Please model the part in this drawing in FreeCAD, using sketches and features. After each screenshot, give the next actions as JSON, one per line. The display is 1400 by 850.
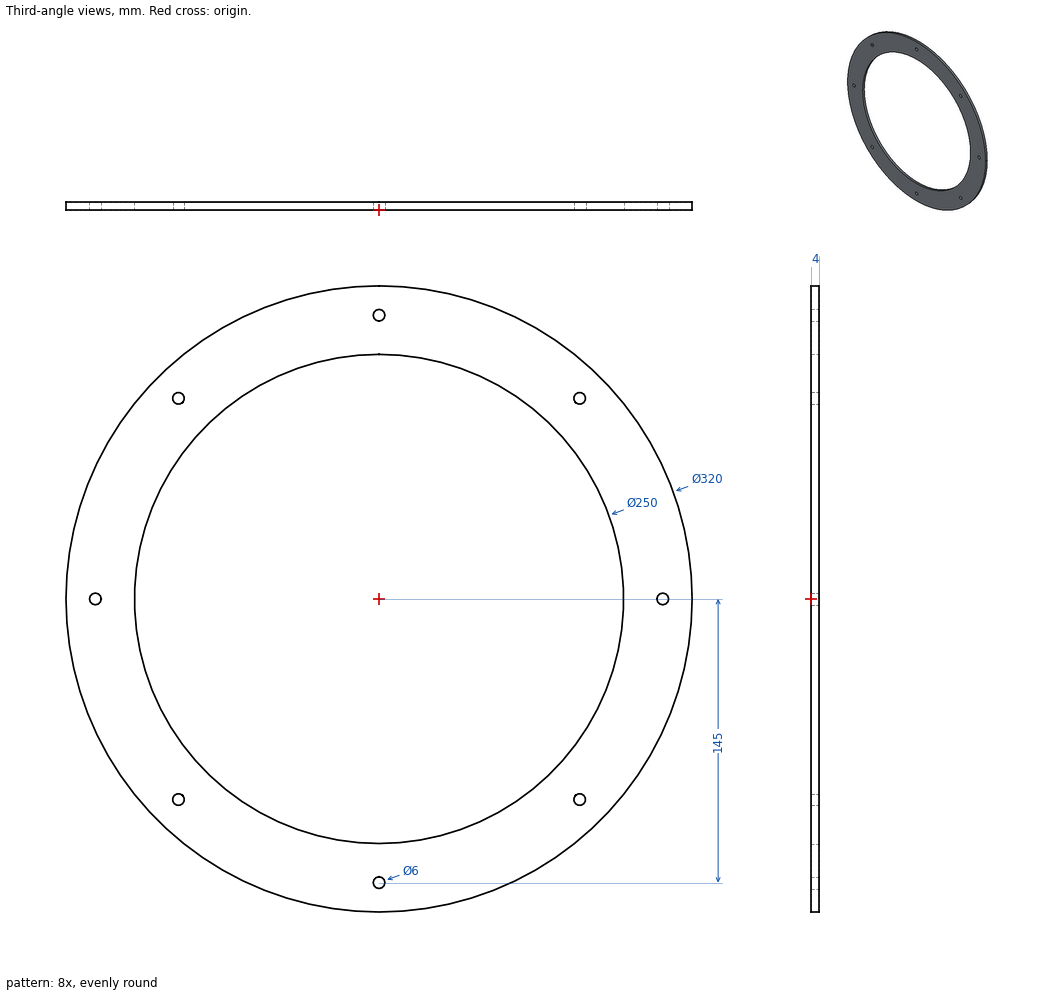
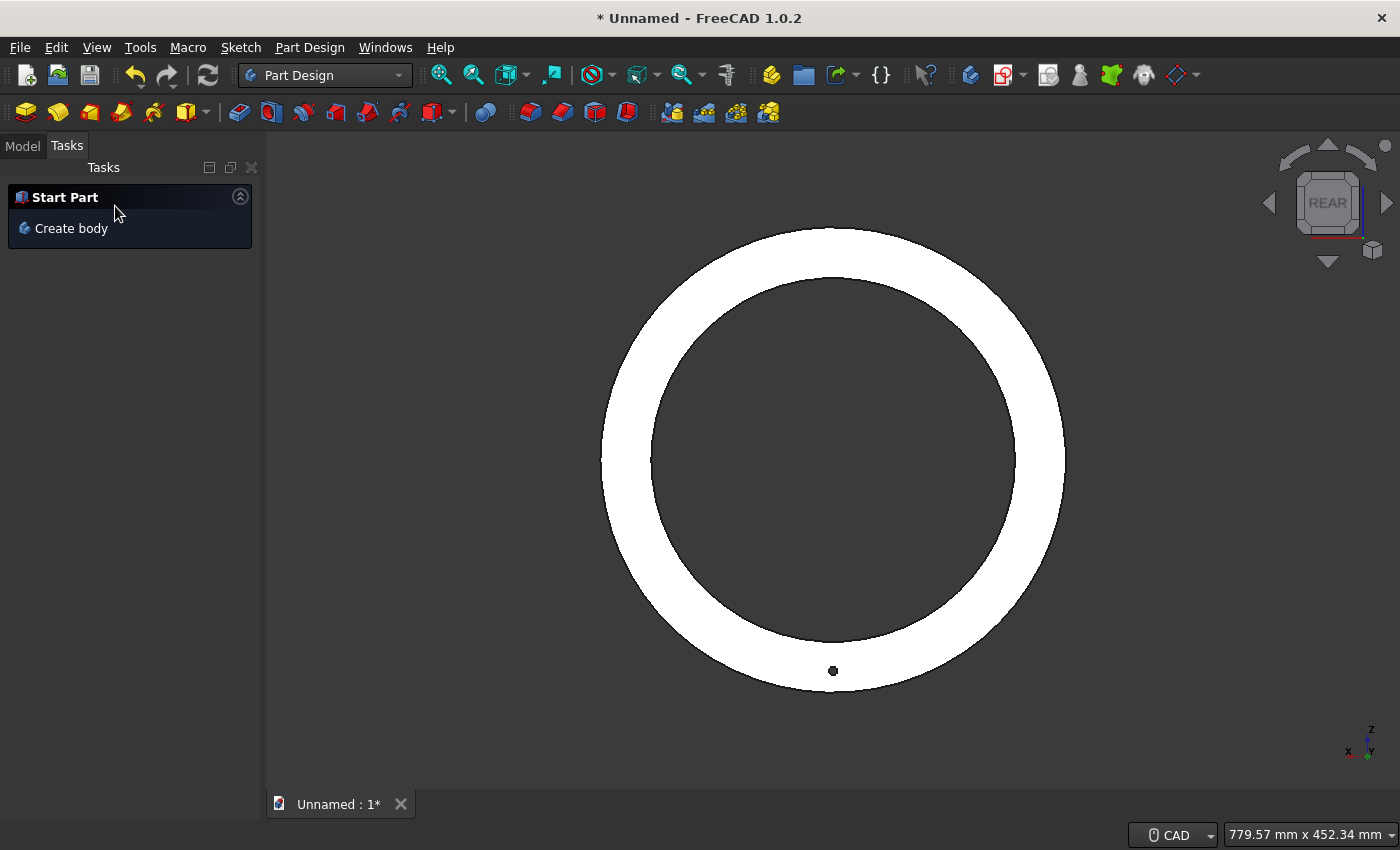
{"action": "left_click", "coordinate": [23, 145]}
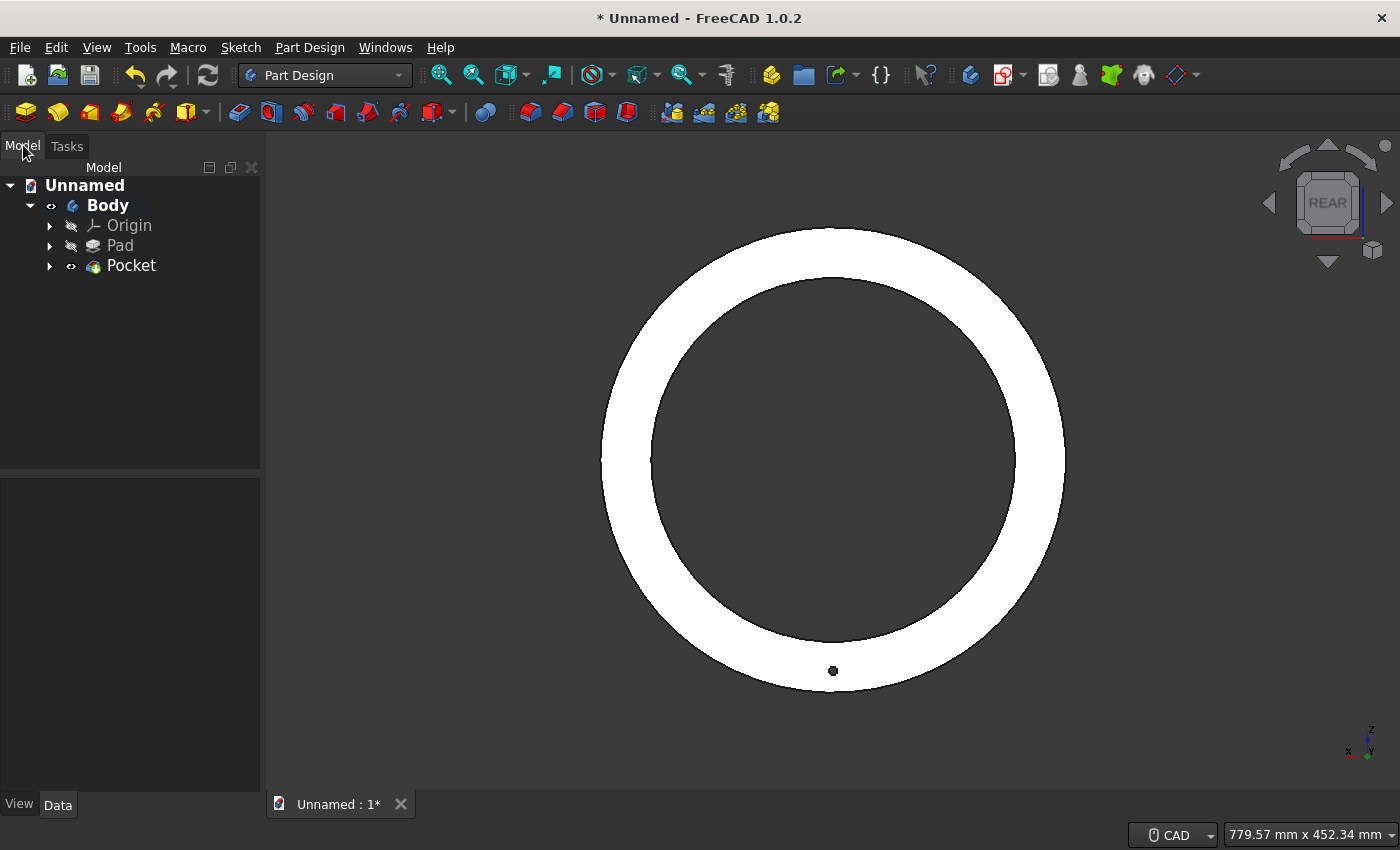
{"action": "left_click", "coordinate": [116, 266]}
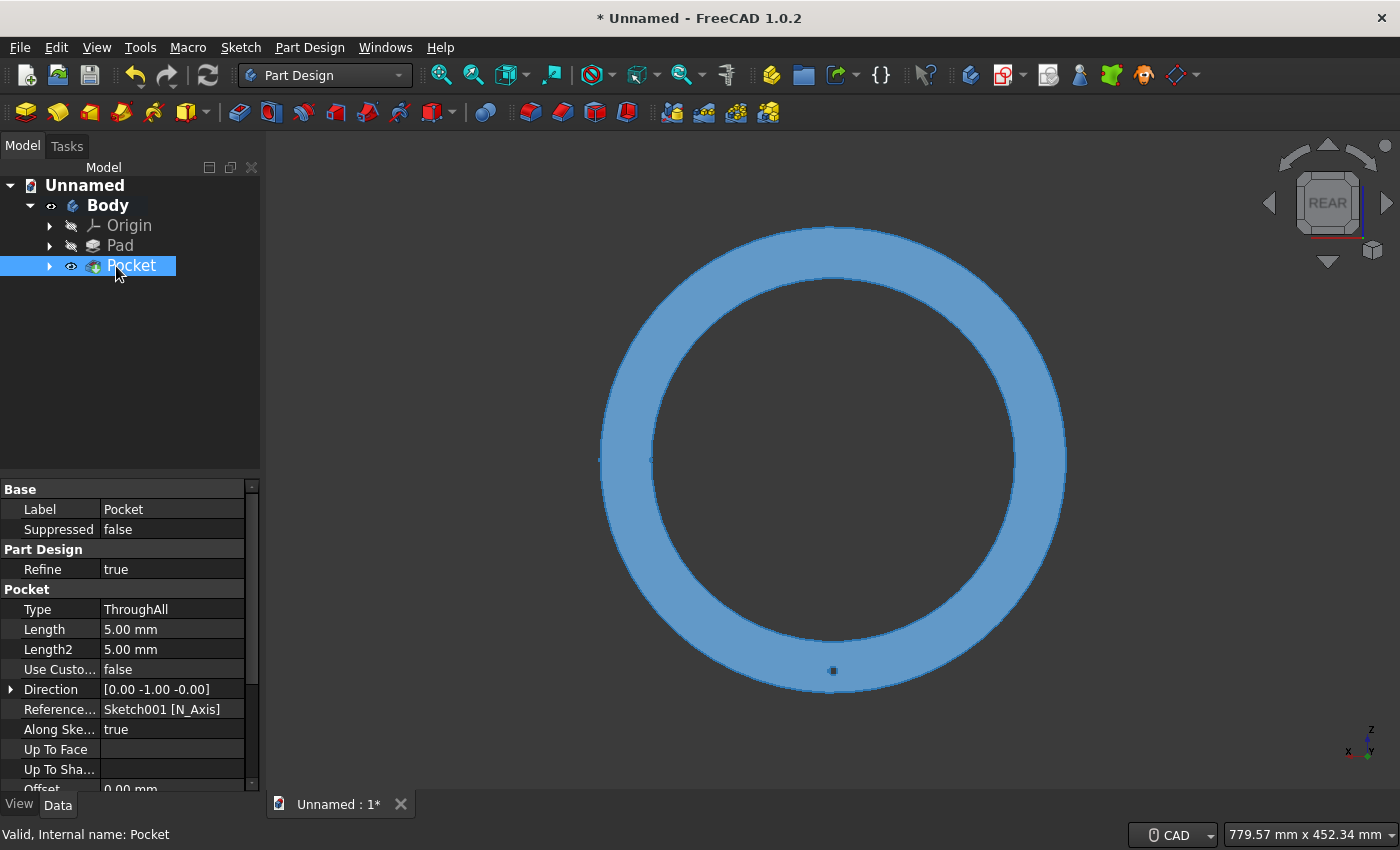
{"action": "left_click", "coordinate": [736, 112]}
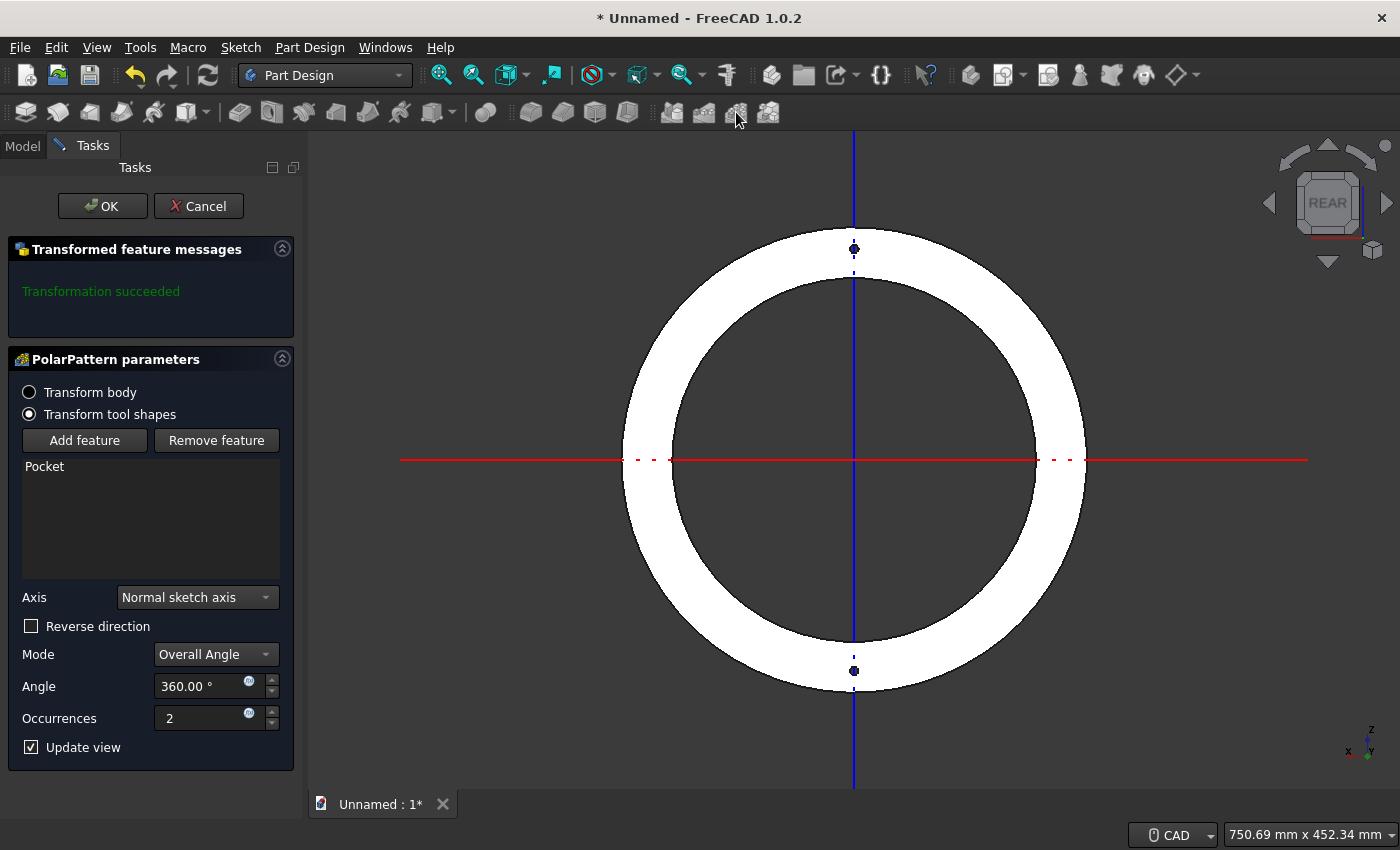
{"action": "left_click", "coordinate": [198, 598]}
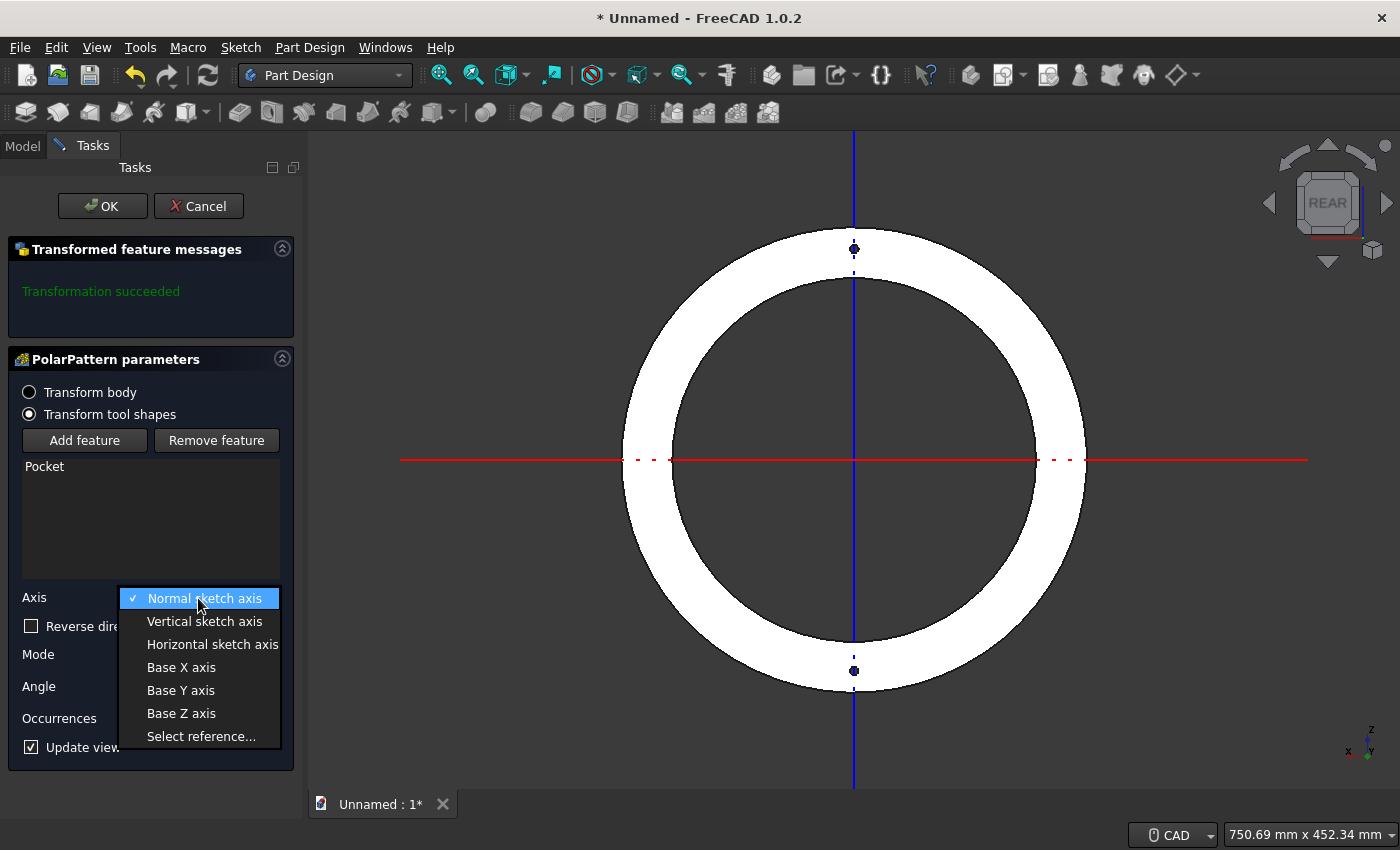
{"action": "left_click", "coordinate": [198, 690]}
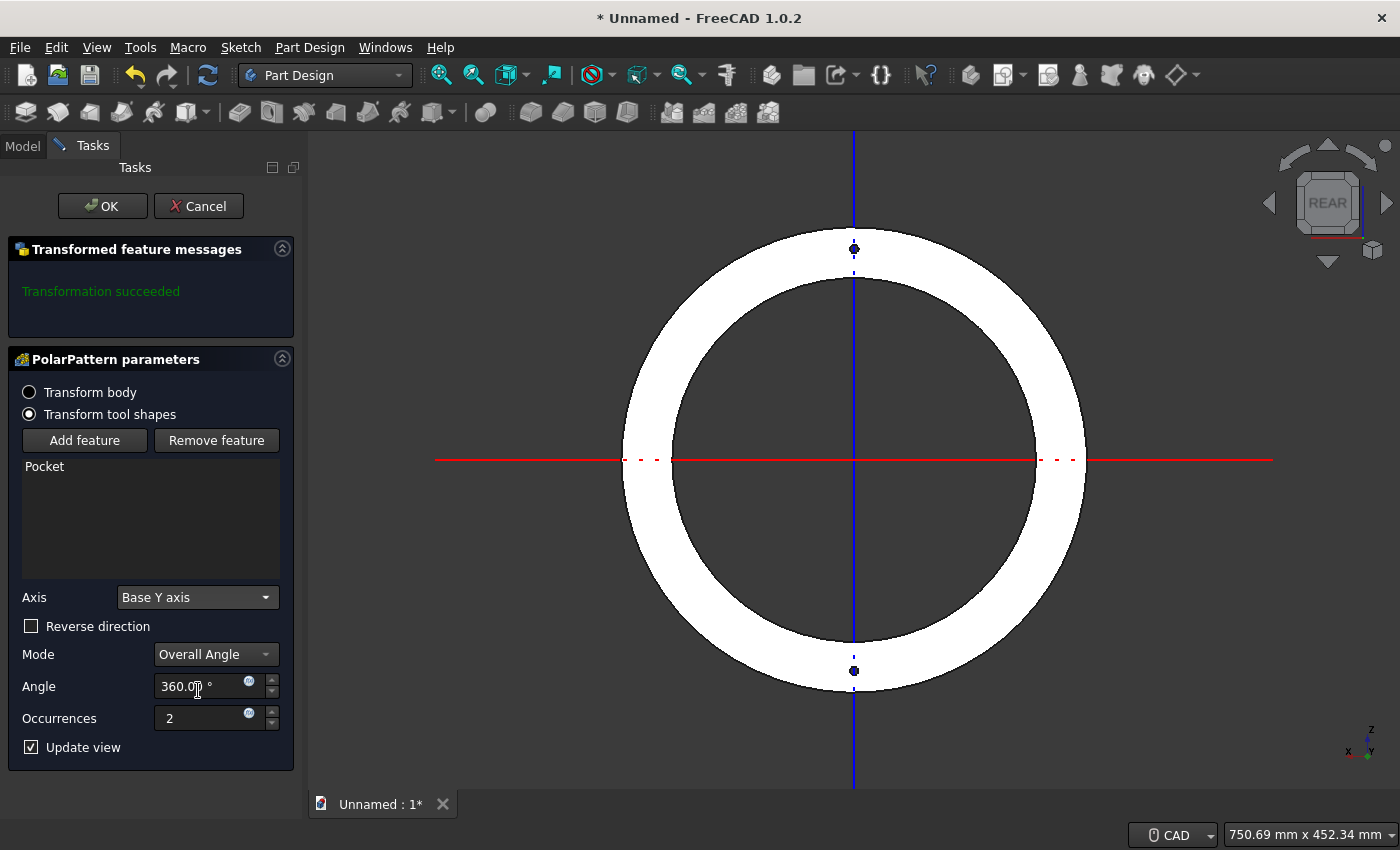
{"action": "triple_click", "coordinate": [209, 718]}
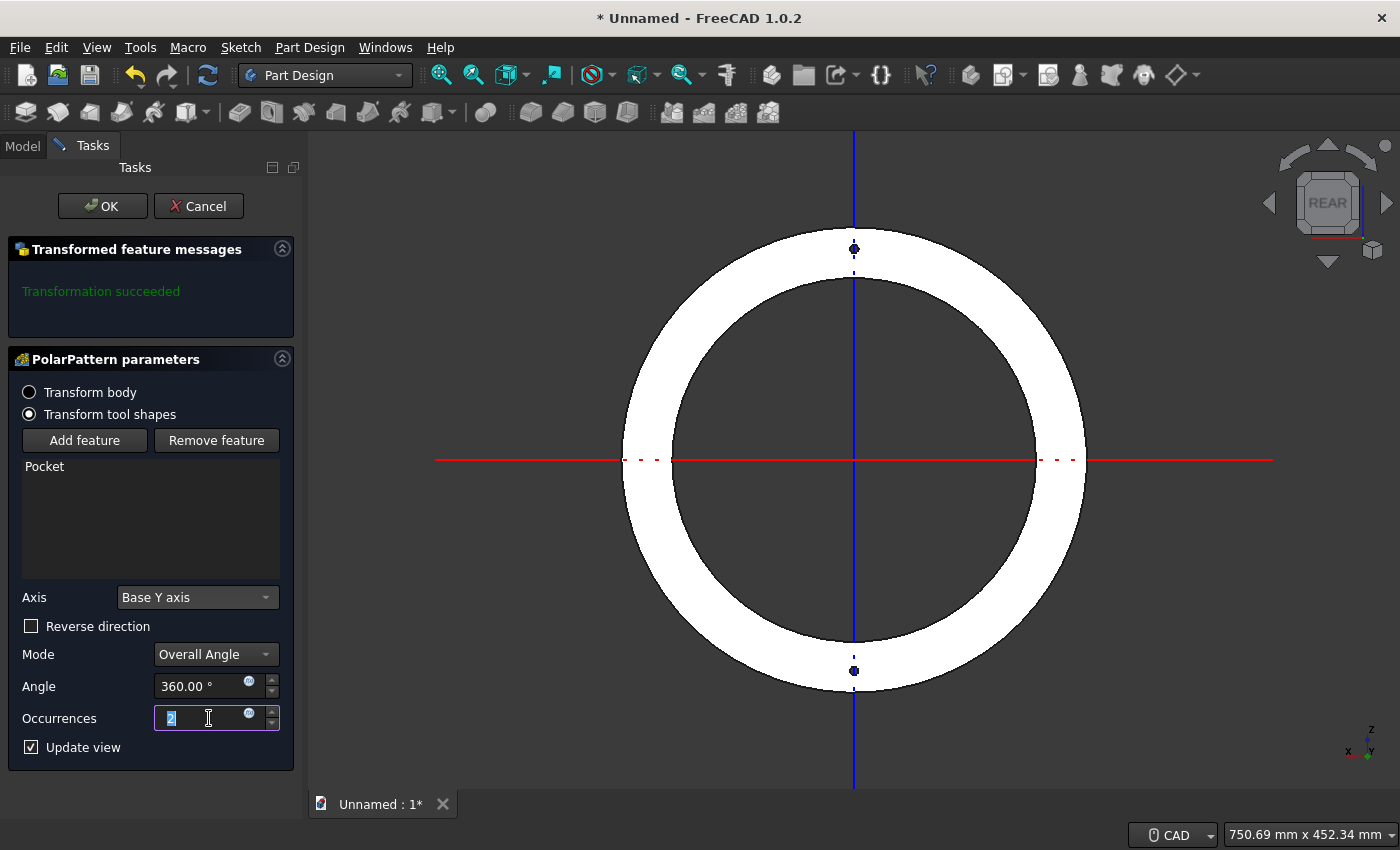
{"action": "type", "text": "8"}
{"action": "key", "text": "Tab"}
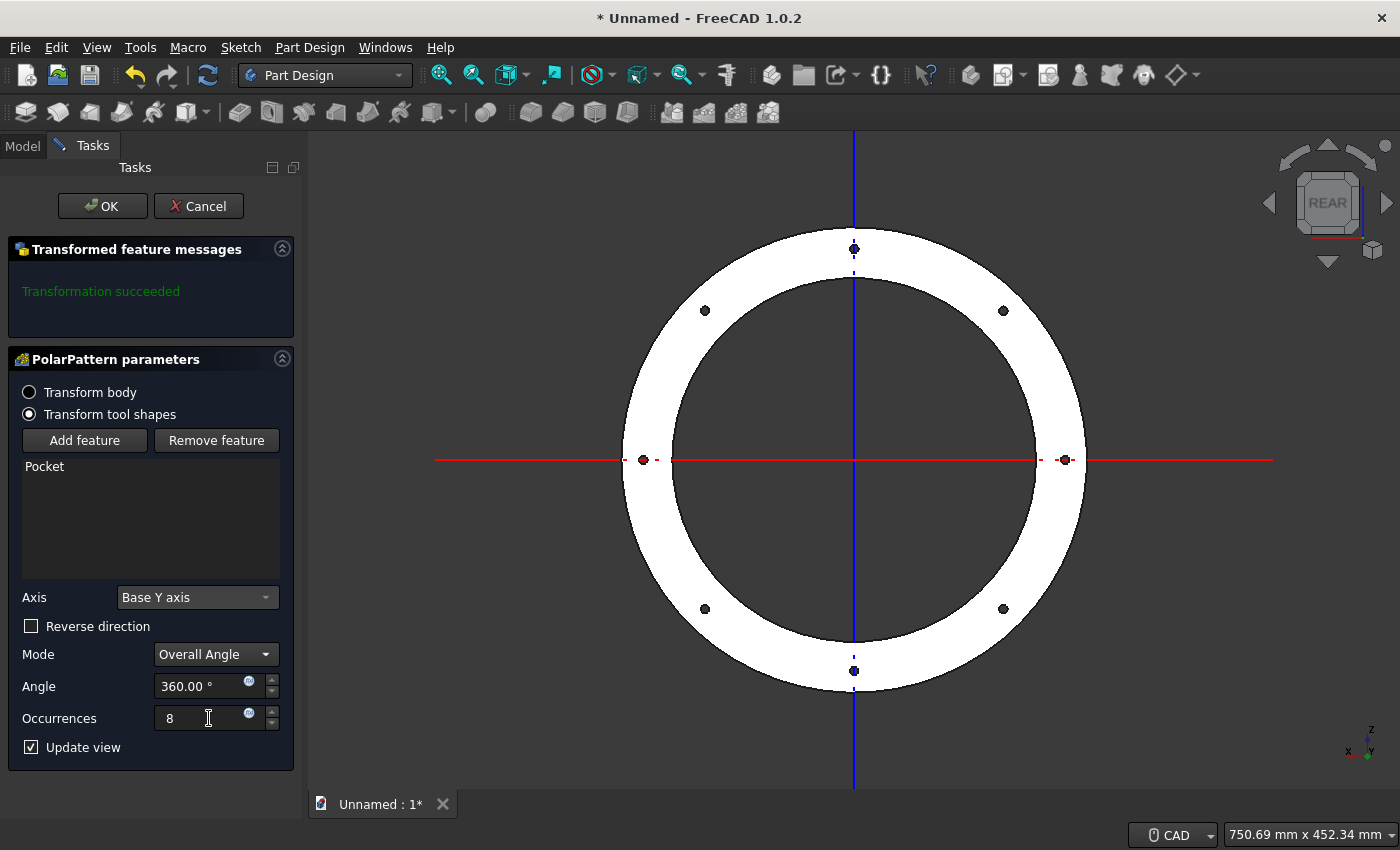
{"action": "left_click", "coordinate": [103, 206]}